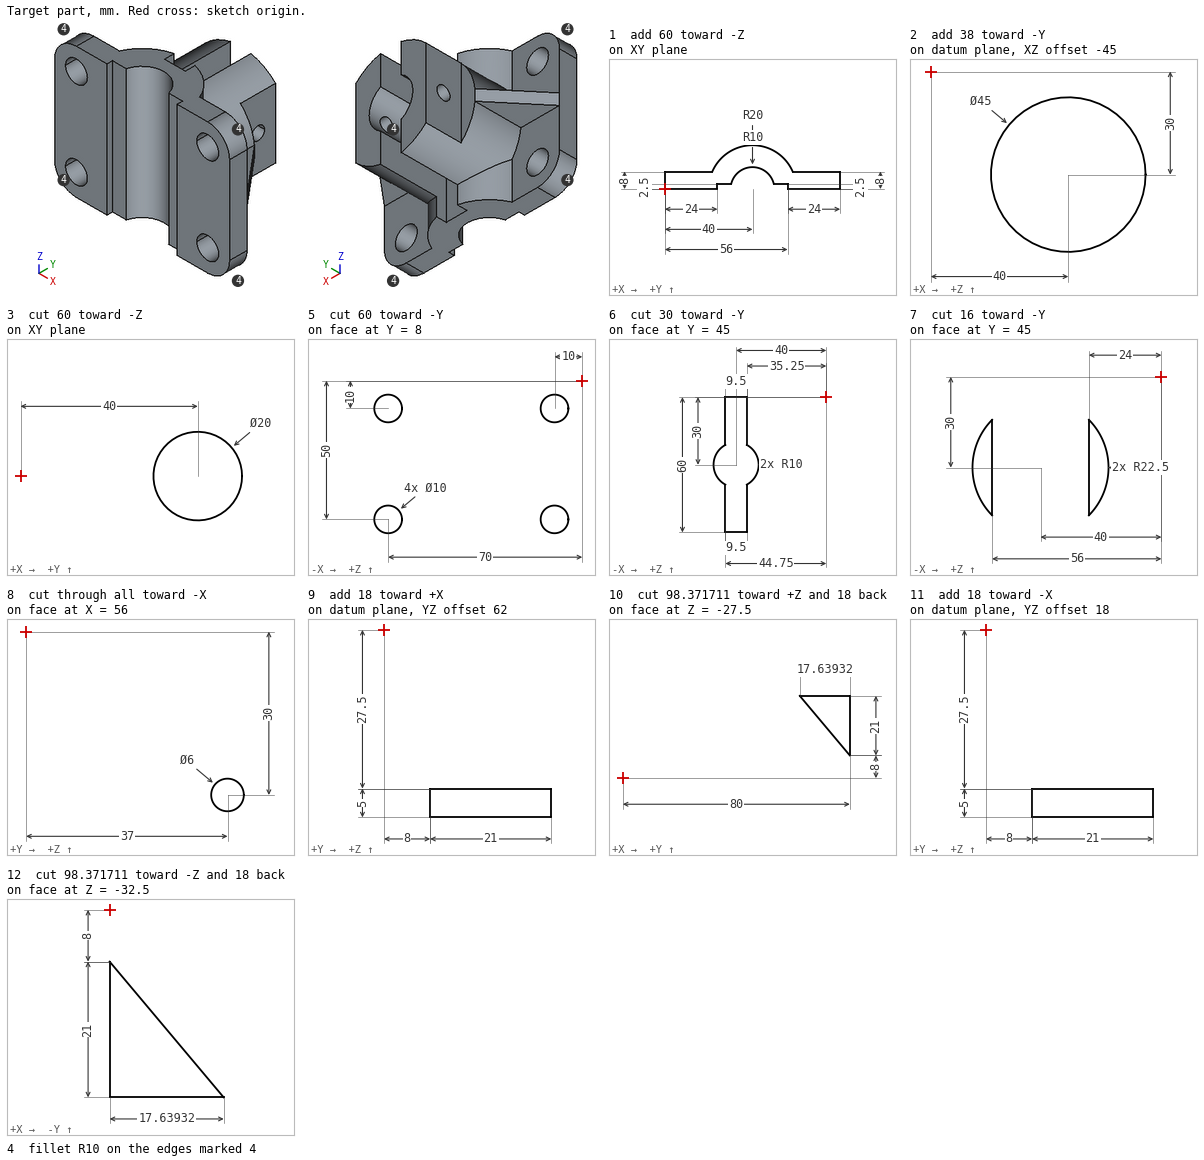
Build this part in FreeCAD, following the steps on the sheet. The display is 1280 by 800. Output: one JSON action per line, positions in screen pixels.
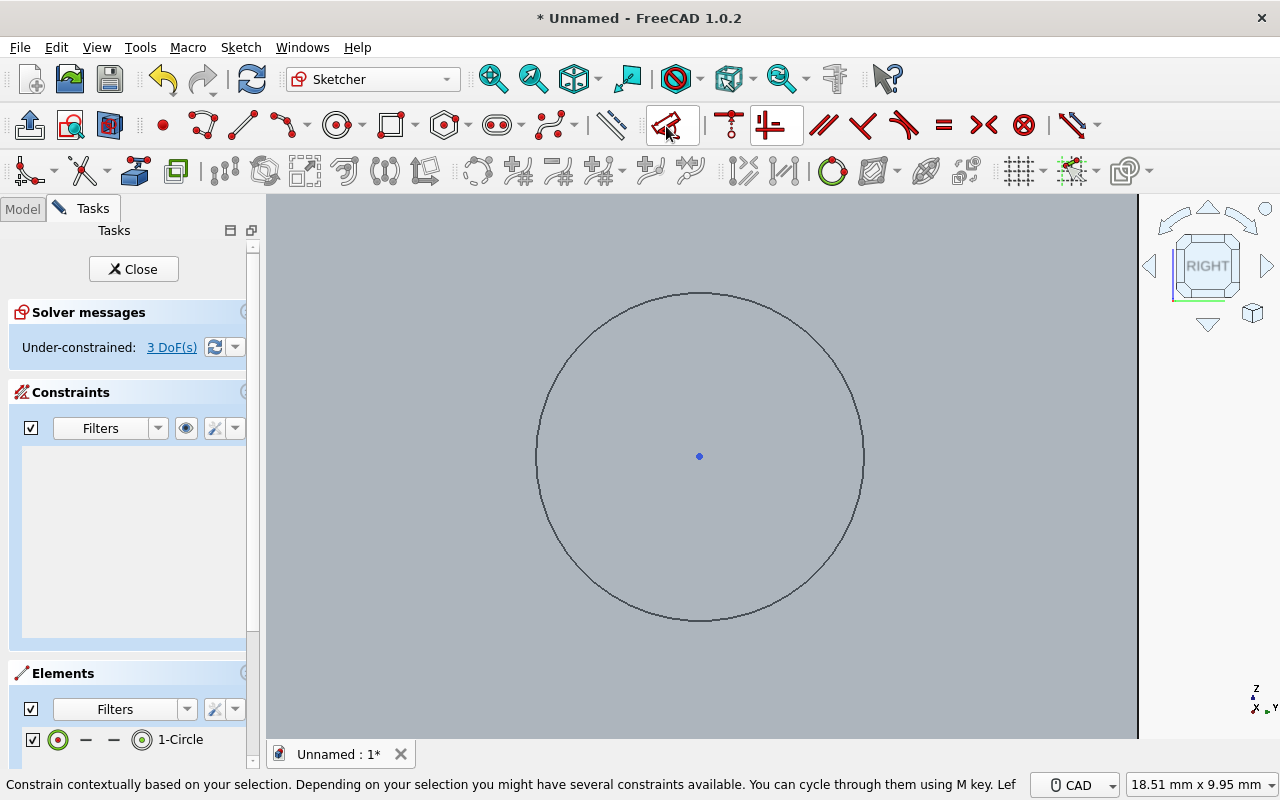
{"action": "left_click", "coordinate": [816, 341]}
{"action": "left_click", "coordinate": [839, 318]}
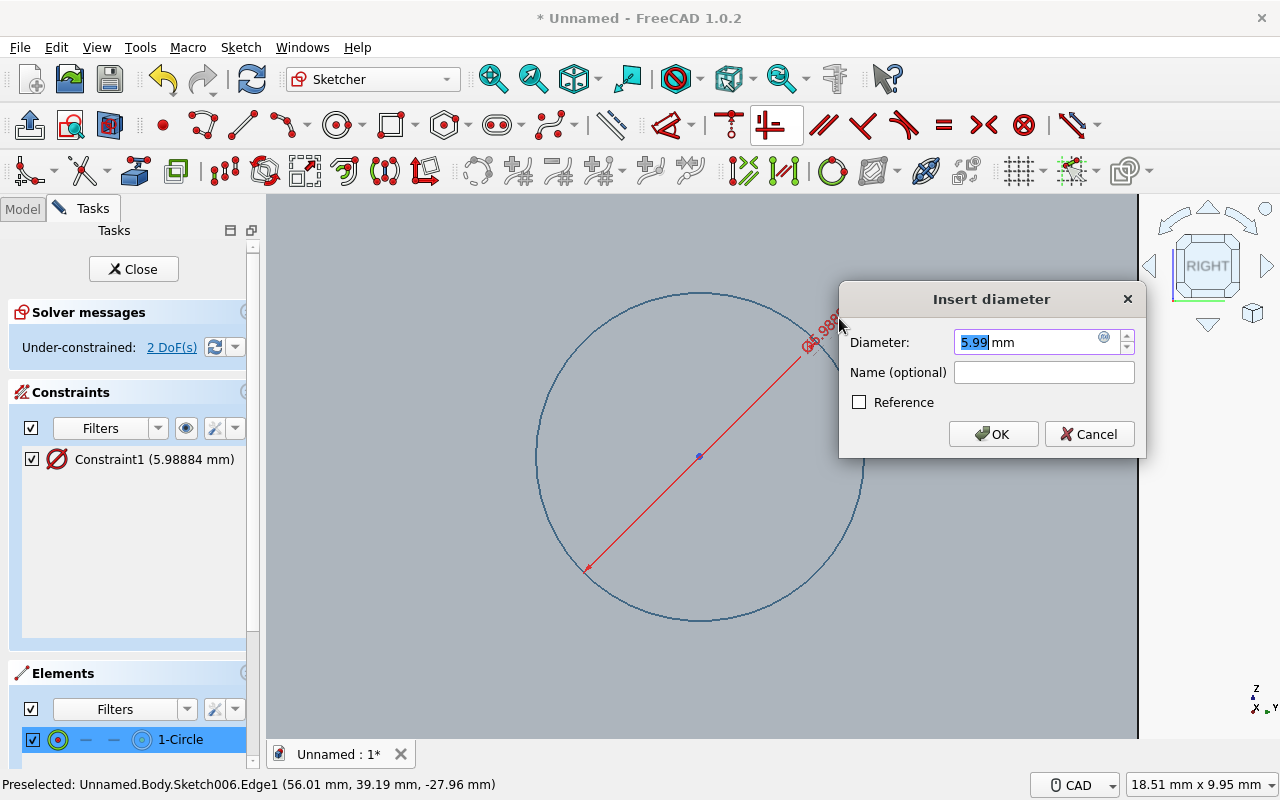
{"action": "type", "text": "6"}
{"action": "key", "text": "Return"}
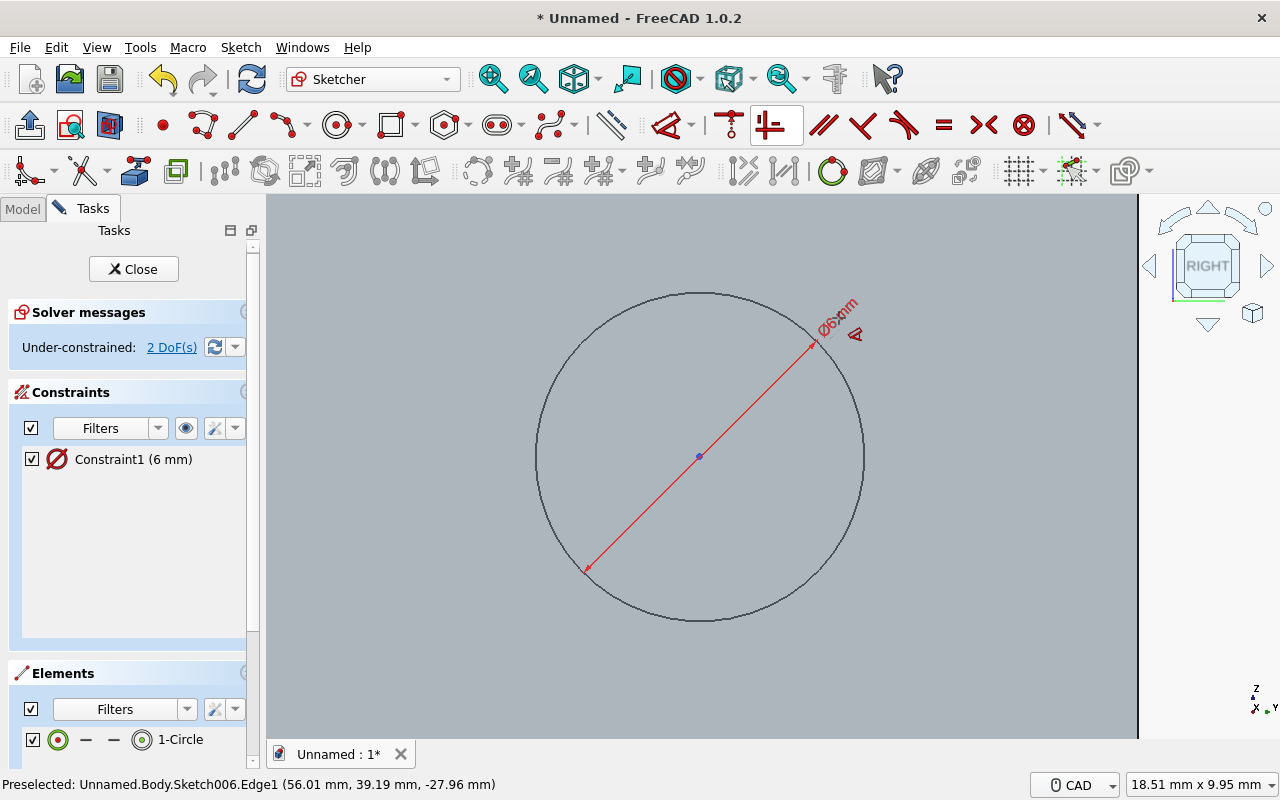
{"action": "left_click", "coordinate": [700, 457]}
{"action": "left_click", "coordinate": [497, 491]}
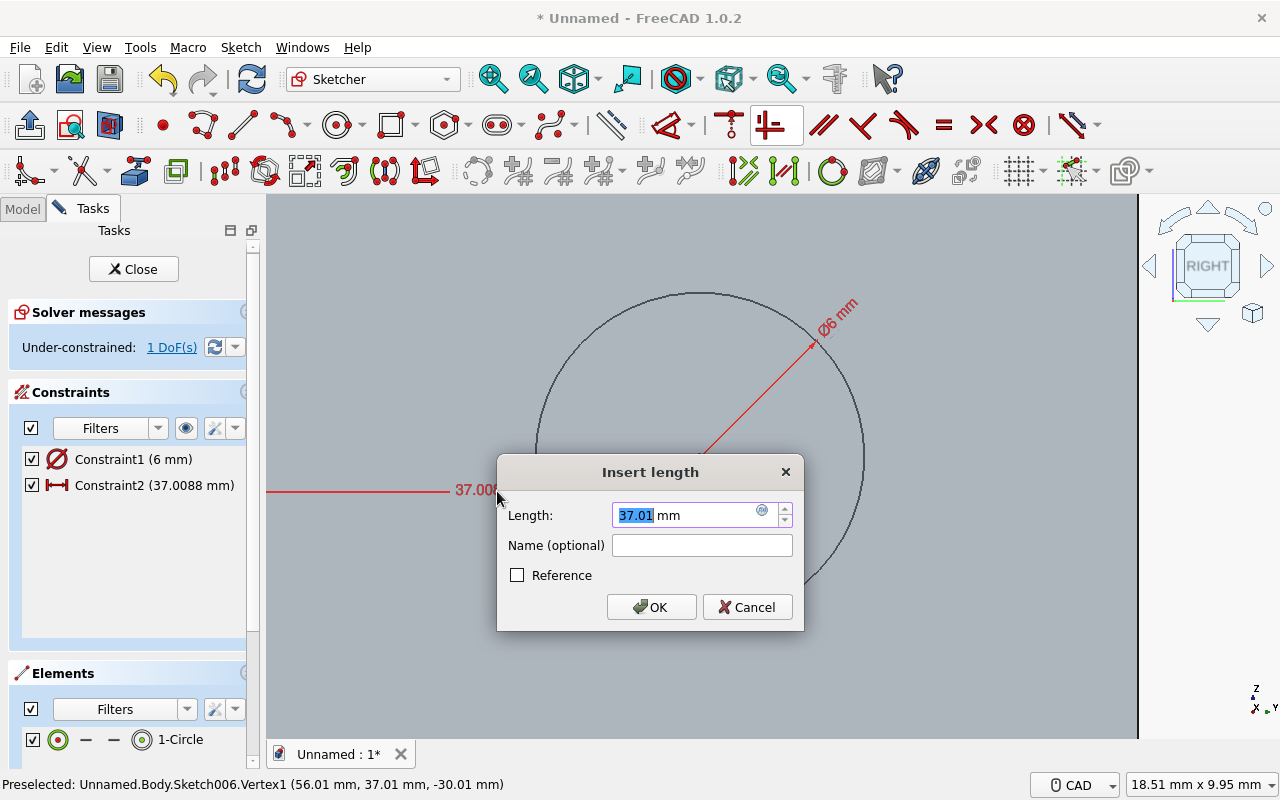
{"action": "type", "text": "37"}
{"action": "key", "text": "Return"}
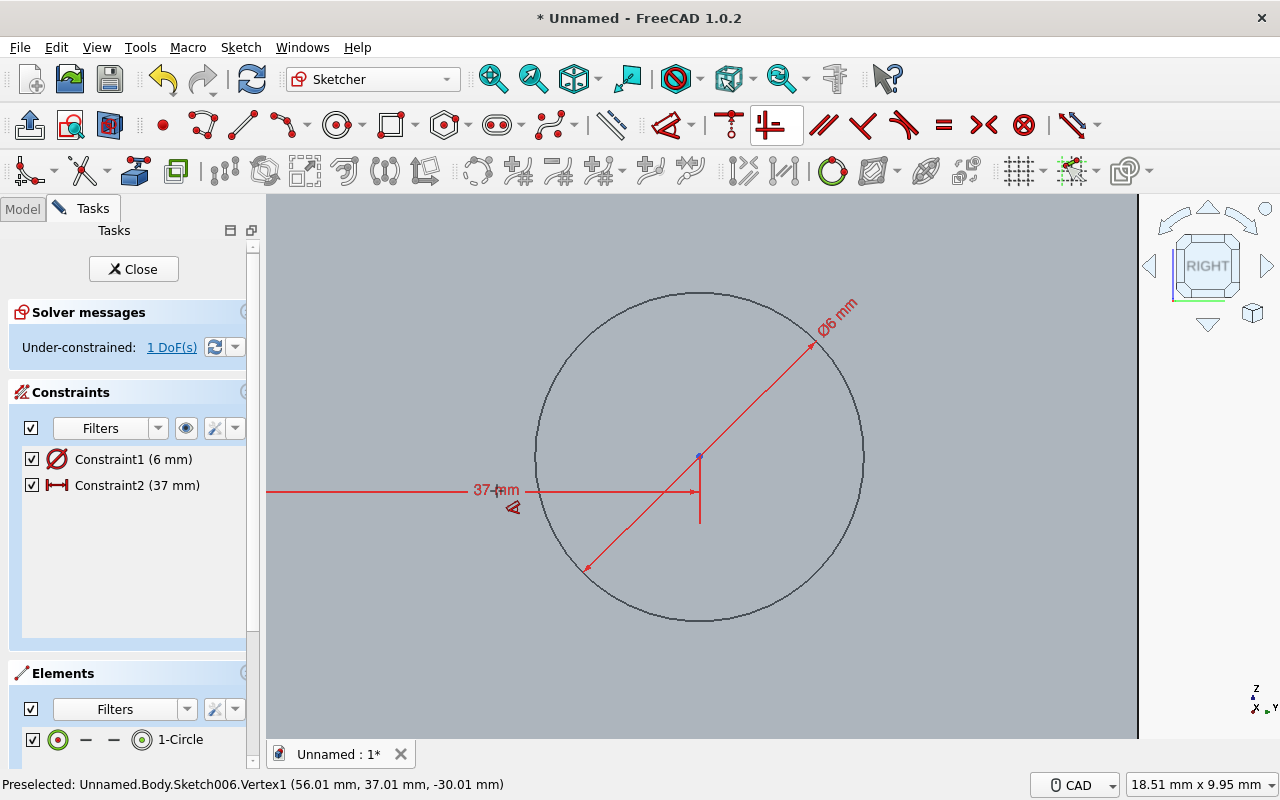
{"action": "left_click", "coordinate": [700, 457]}
{"action": "left_click", "coordinate": [734, 340]}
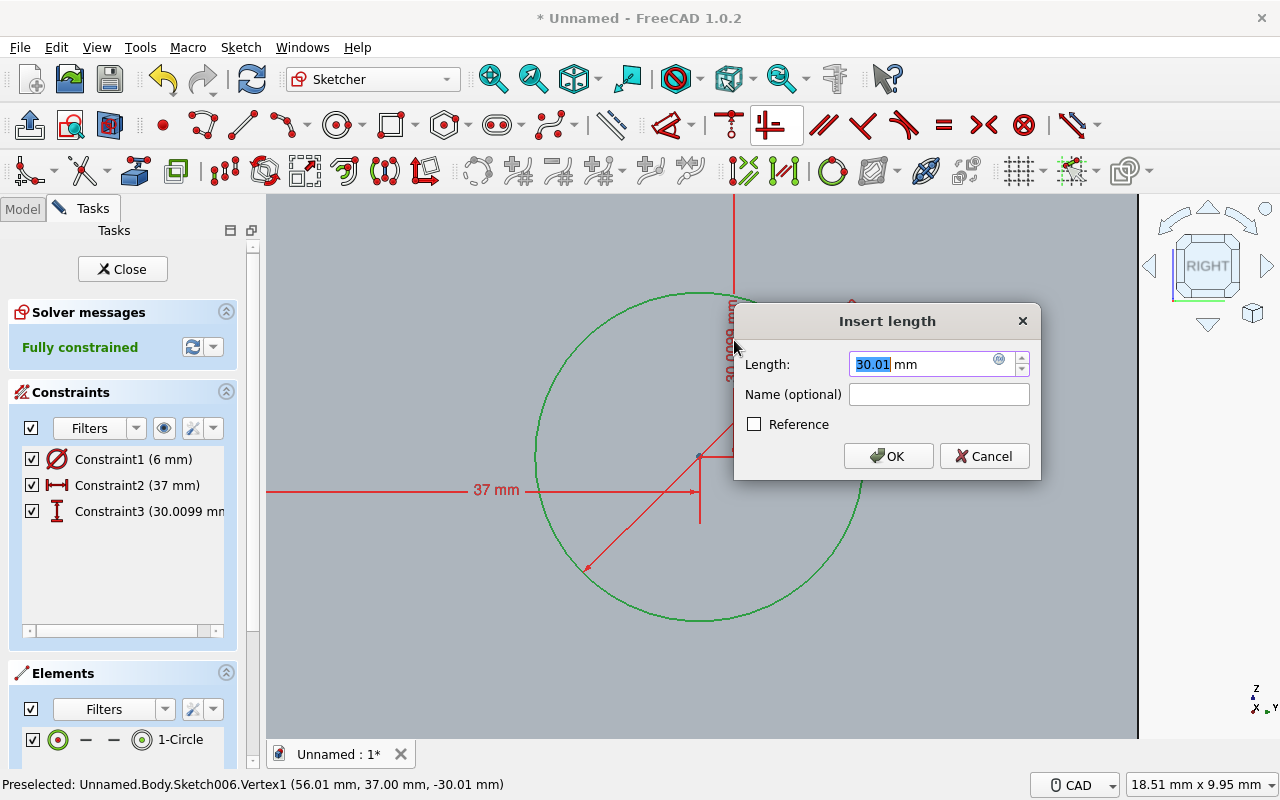
{"action": "type", "text": "30"}
{"action": "key", "text": "Return"}
{"action": "key", "text": "Escape"}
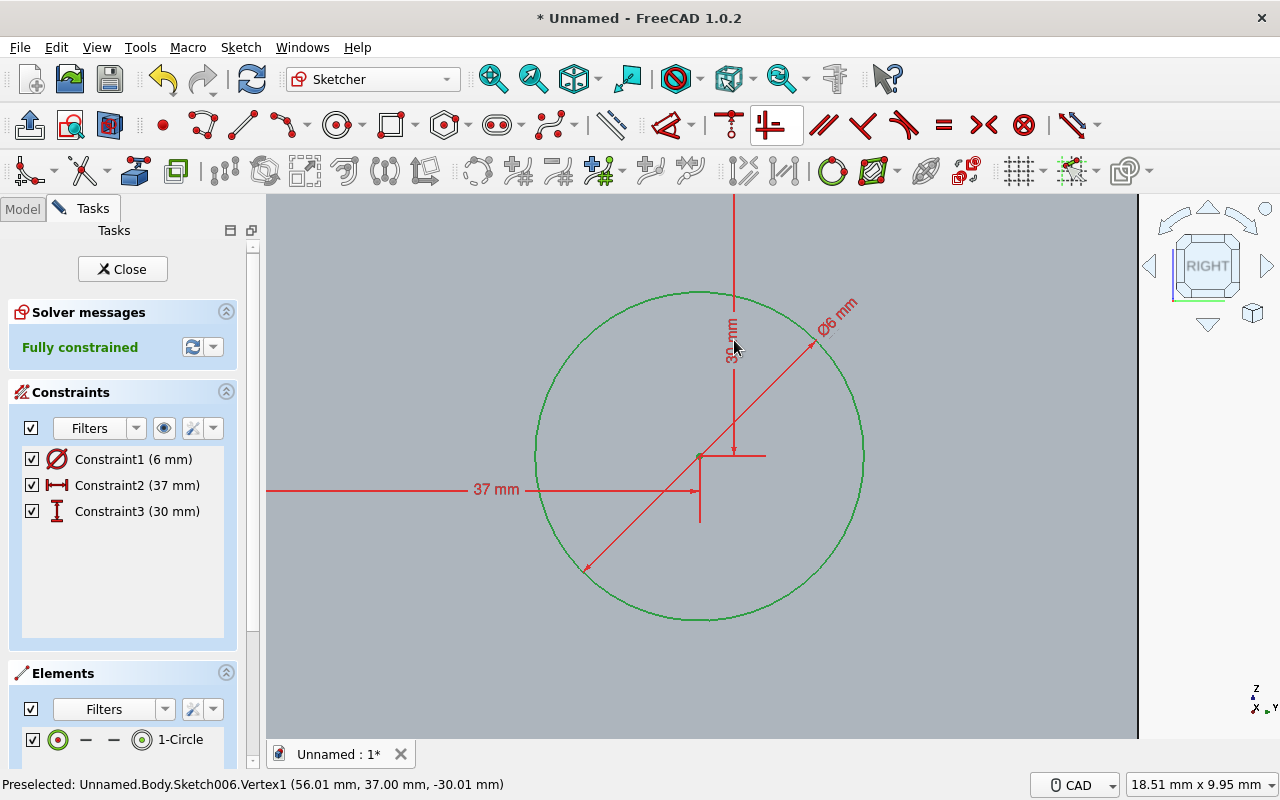
{"action": "left_click", "coordinate": [123, 269]}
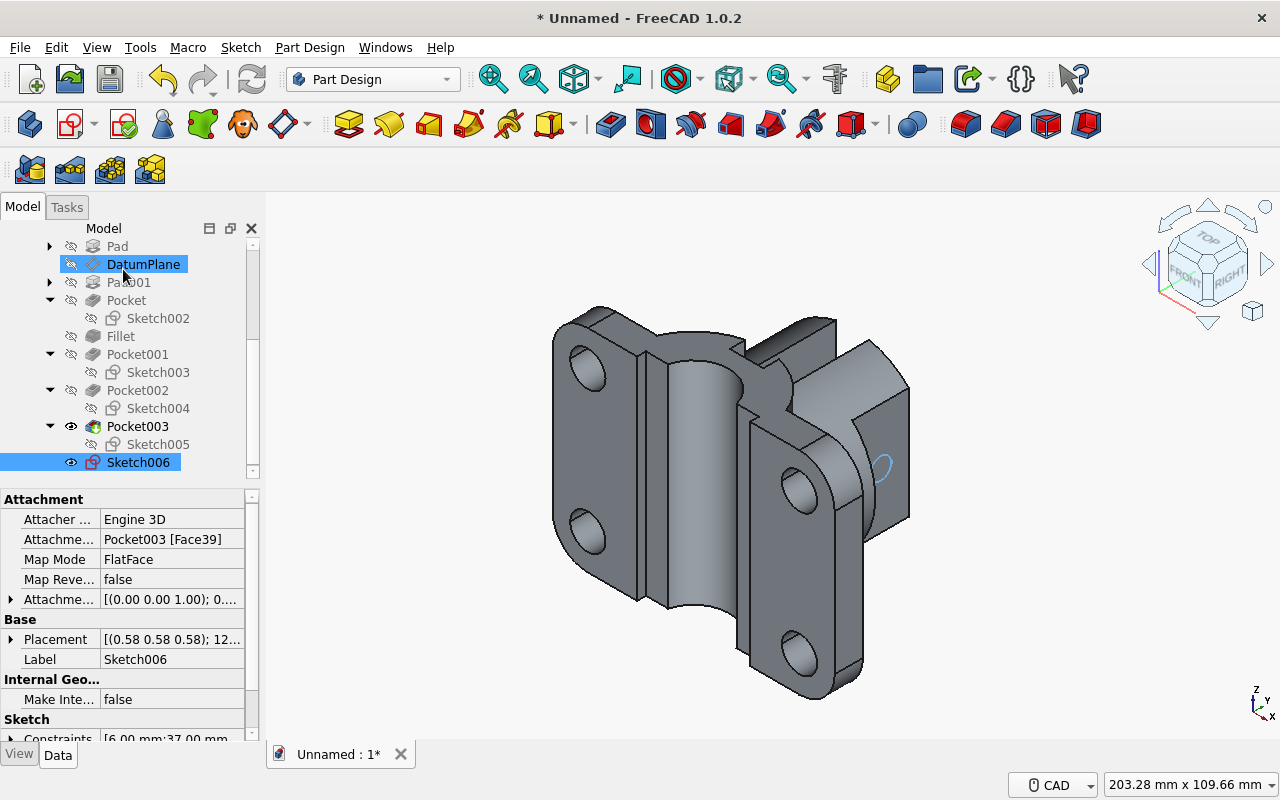
{"action": "left_click", "coordinate": [612, 124]}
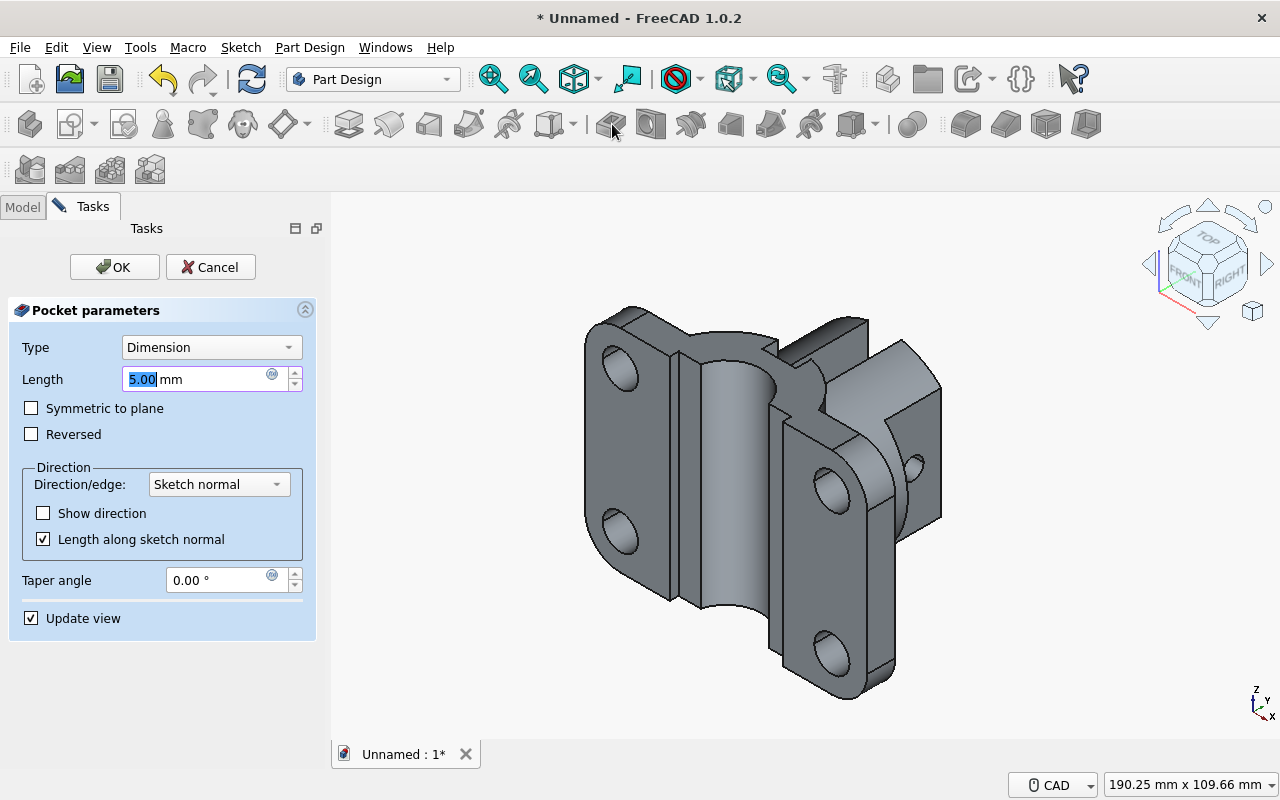
{"action": "left_click", "coordinate": [212, 348]}